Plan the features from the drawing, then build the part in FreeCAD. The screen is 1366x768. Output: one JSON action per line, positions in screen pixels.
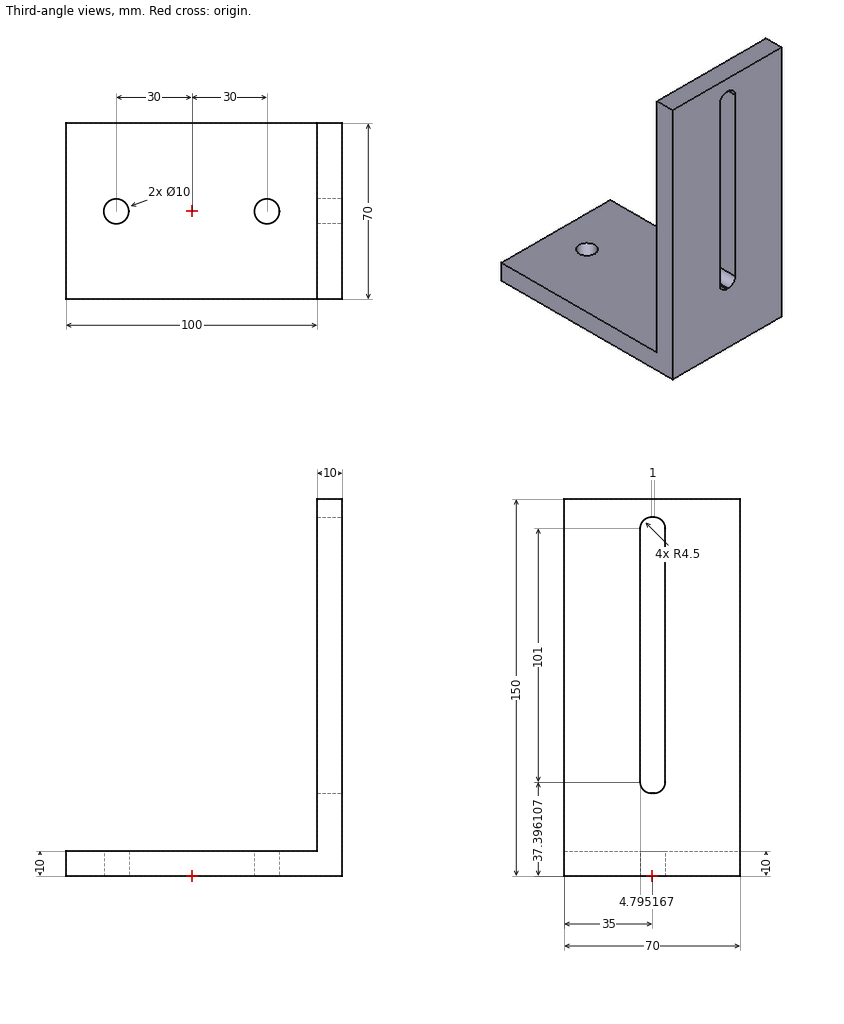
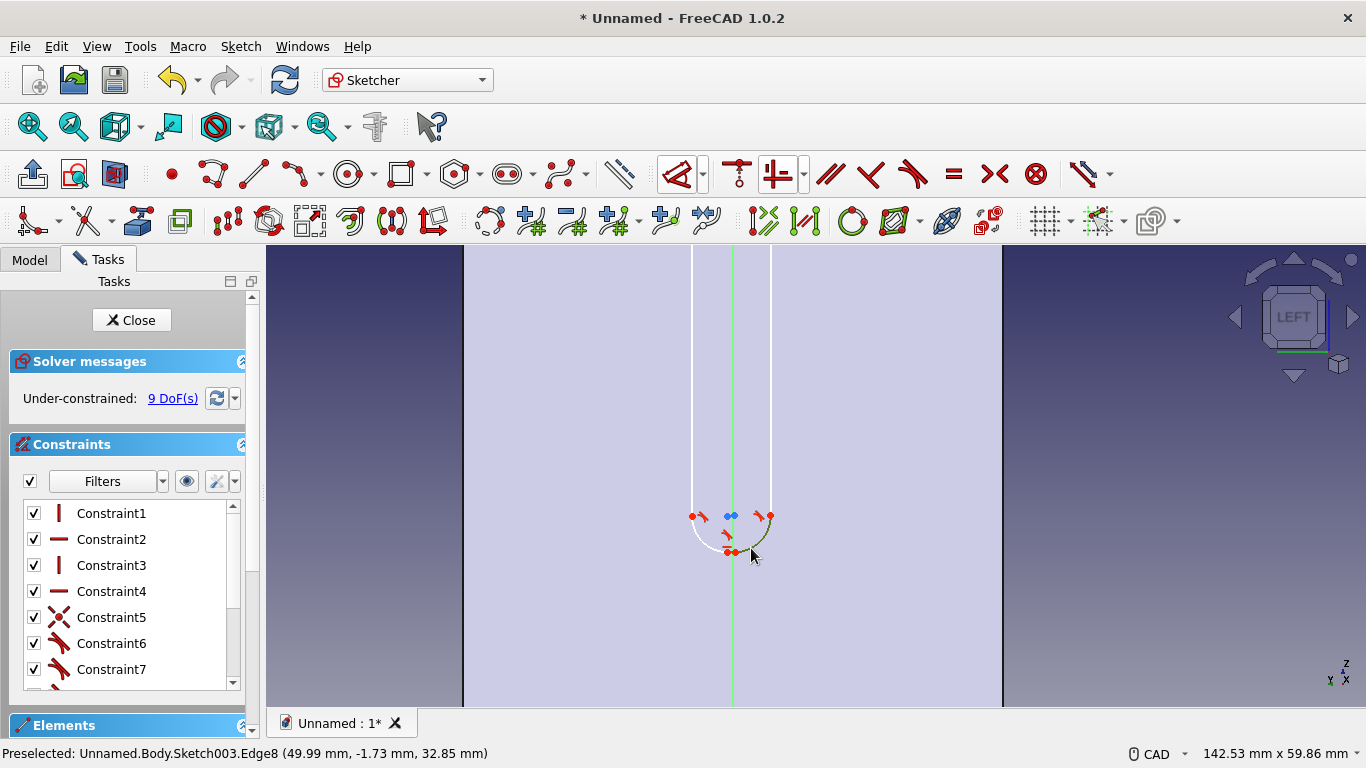
{"action": "left_click", "coordinate": [913, 174]}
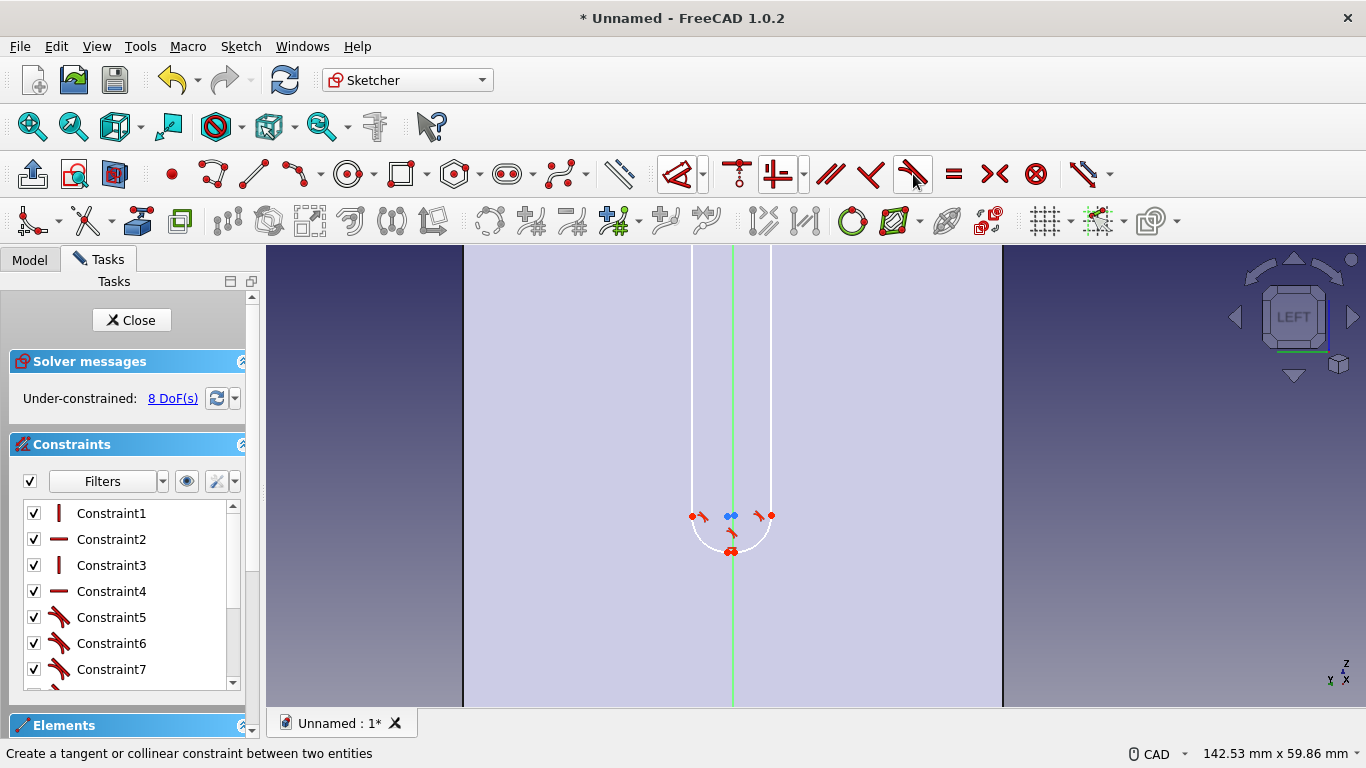
{"action": "scroll", "coordinate": [753, 549], "scroll_direction": "down", "scroll_amount": 7}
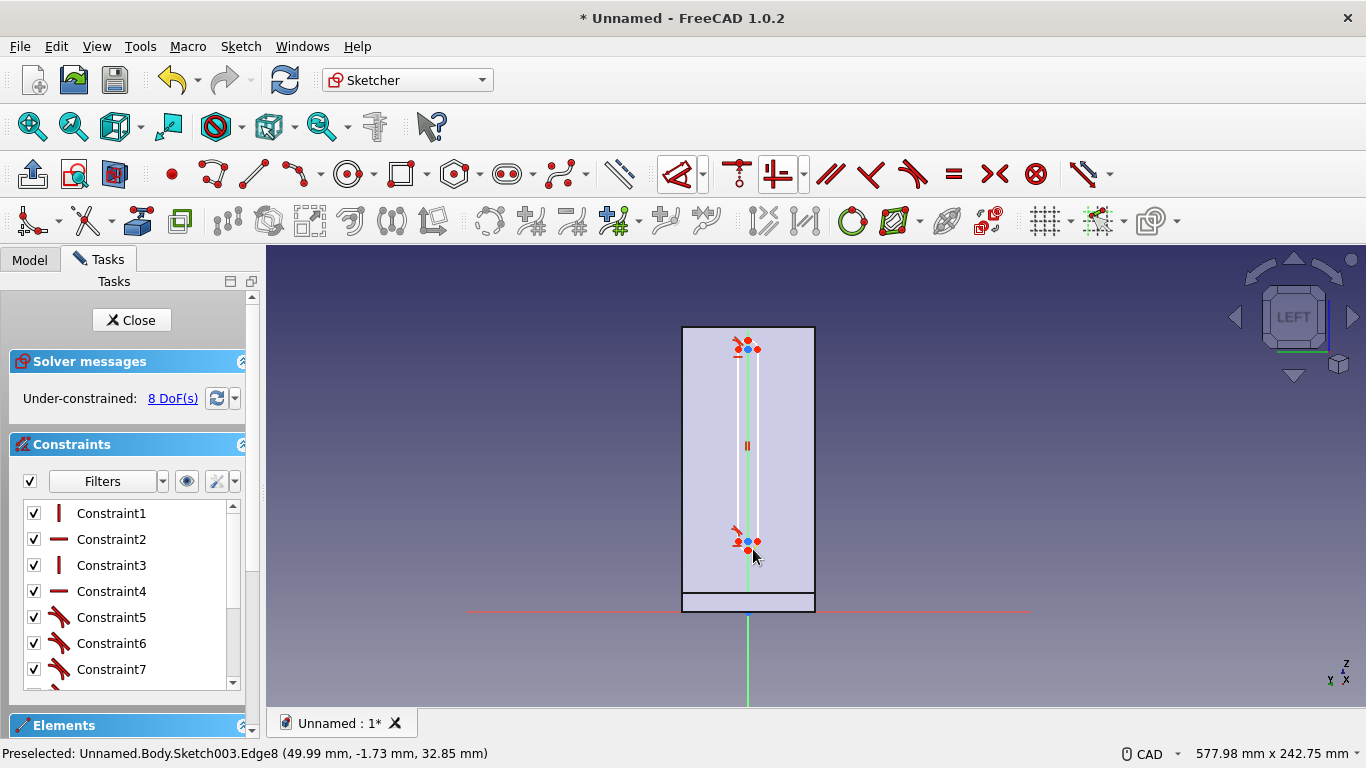
{"action": "scroll", "coordinate": [757, 345], "scroll_direction": "up", "scroll_amount": 6}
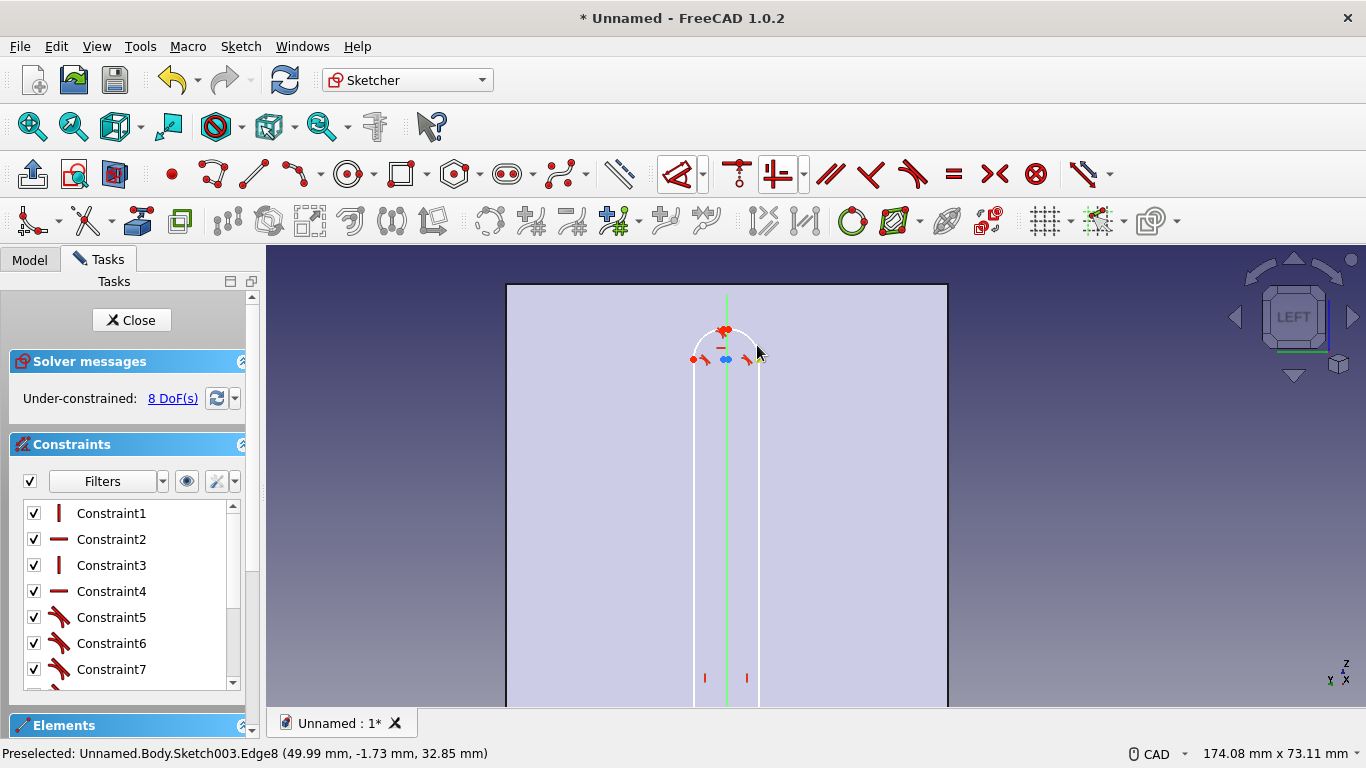
{"action": "left_click", "coordinate": [755, 346]}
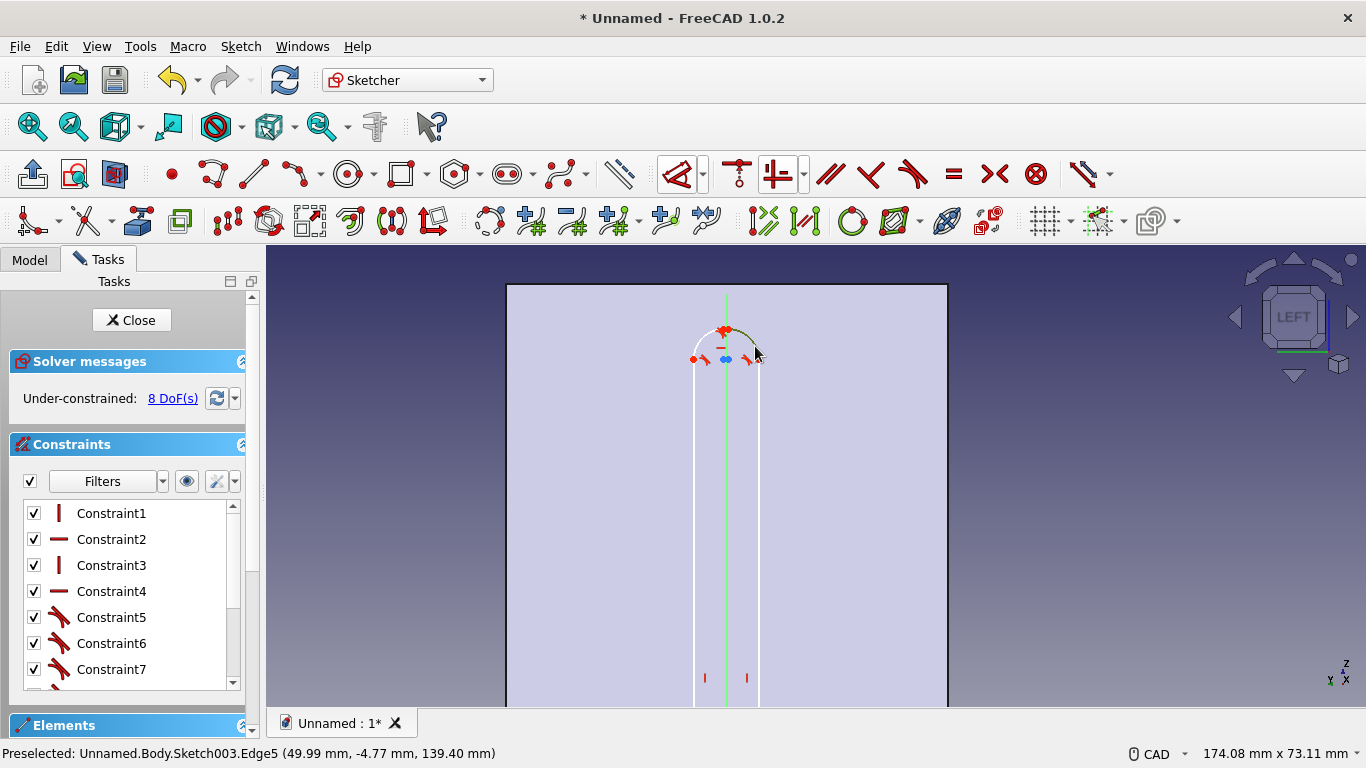
{"action": "left_click", "coordinate": [710, 332]}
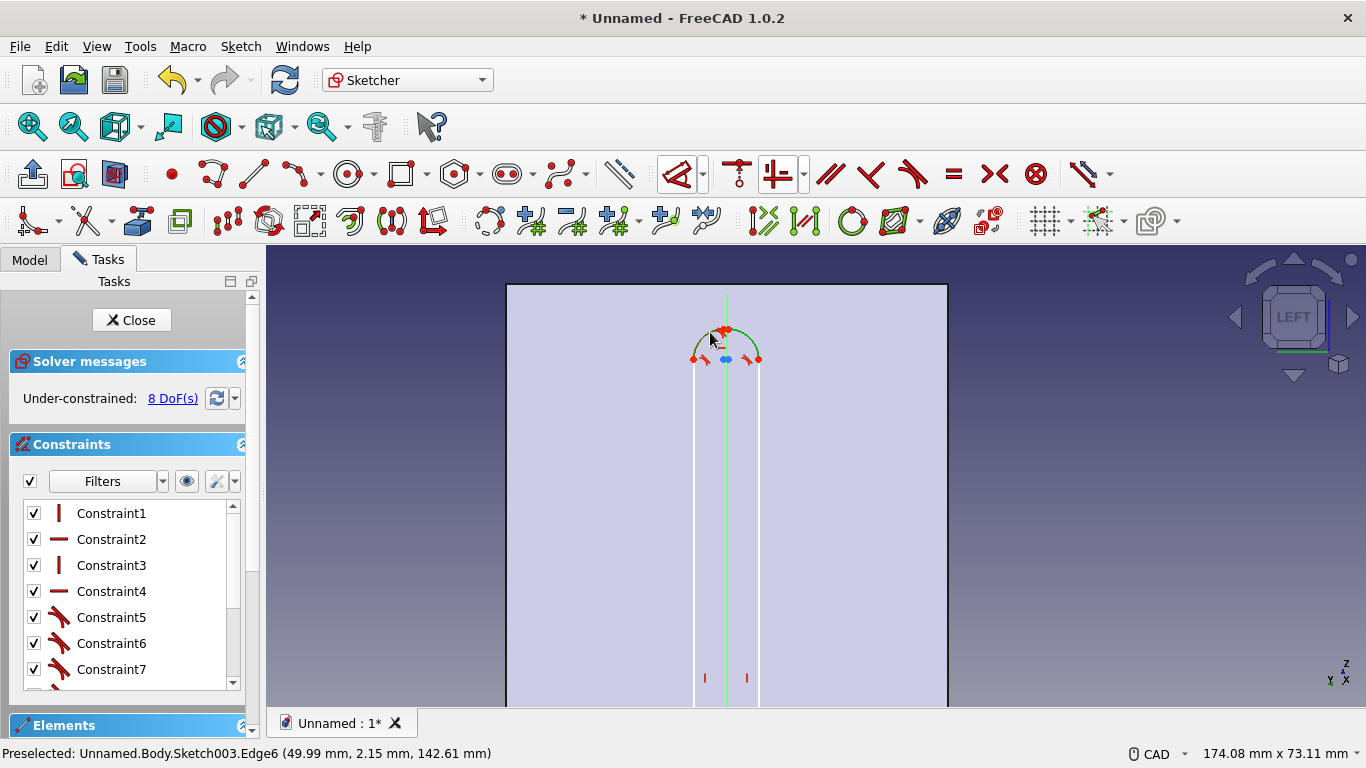
{"action": "scroll", "coordinate": [757, 345], "scroll_direction": "down", "scroll_amount": 6}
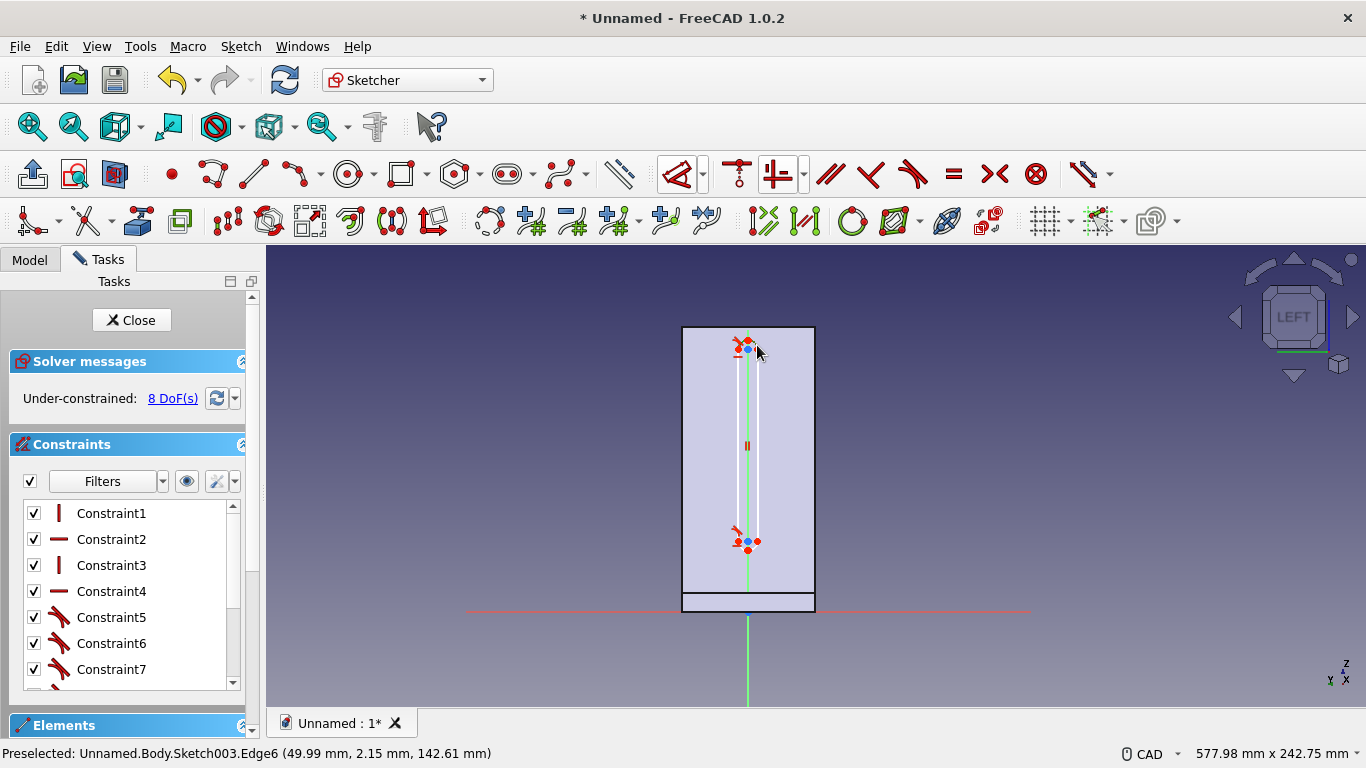
{"action": "scroll", "coordinate": [739, 545], "scroll_direction": "up", "scroll_amount": 7}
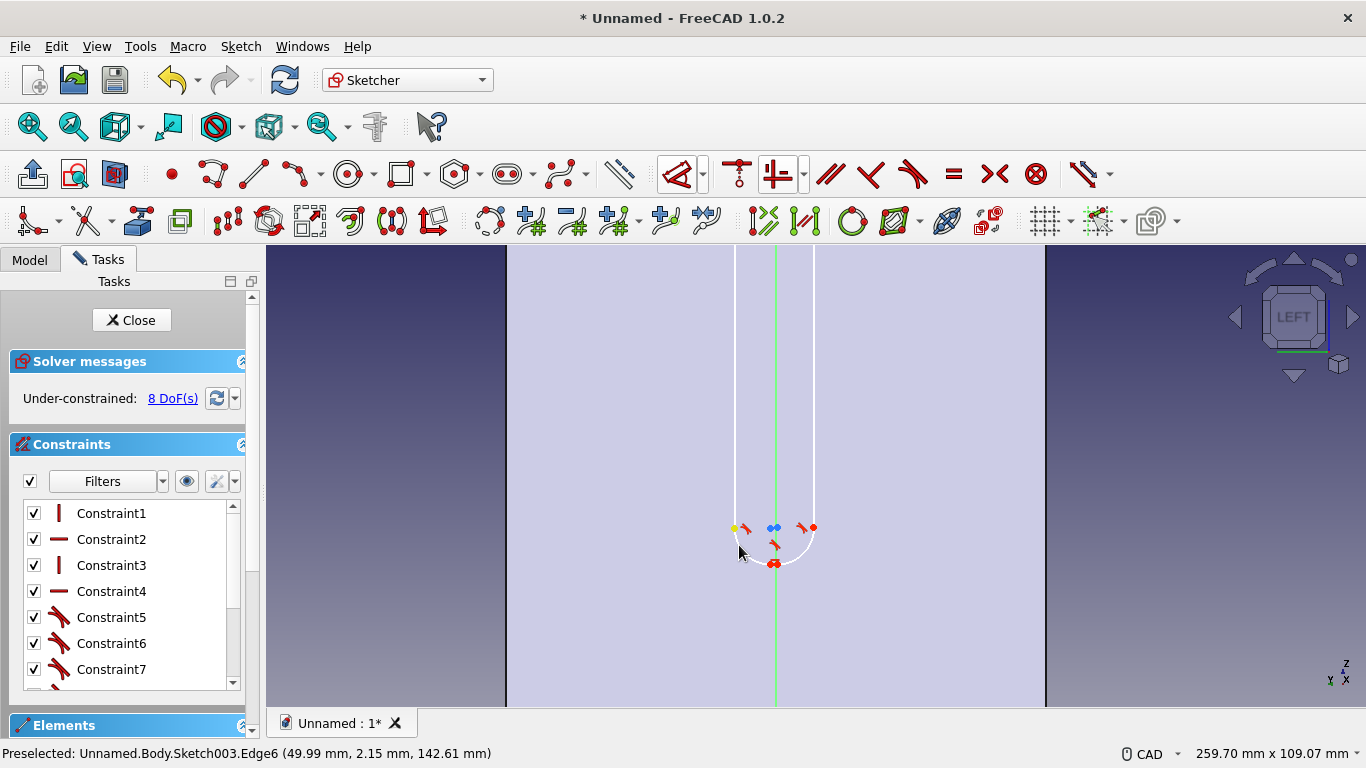
{"action": "left_click", "coordinate": [739, 545]}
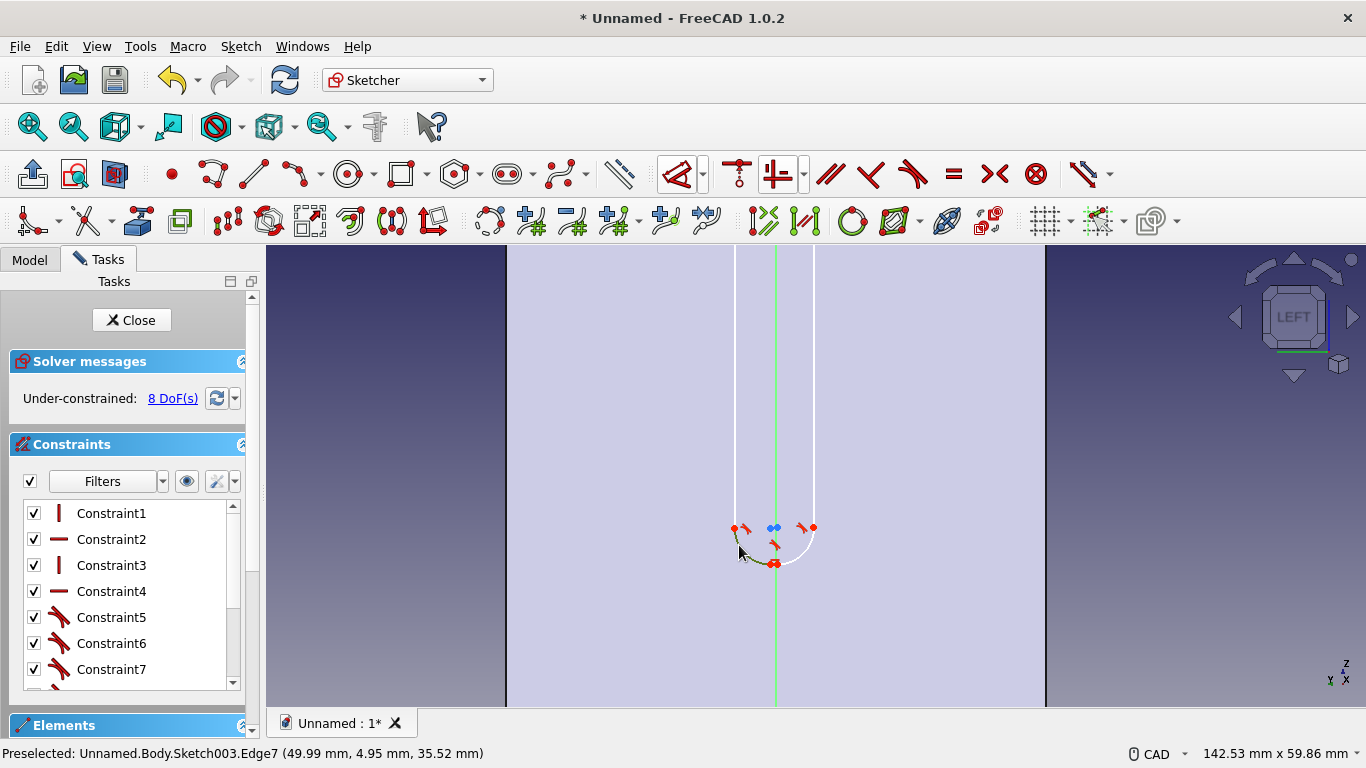
{"action": "left_click", "coordinate": [794, 560]}